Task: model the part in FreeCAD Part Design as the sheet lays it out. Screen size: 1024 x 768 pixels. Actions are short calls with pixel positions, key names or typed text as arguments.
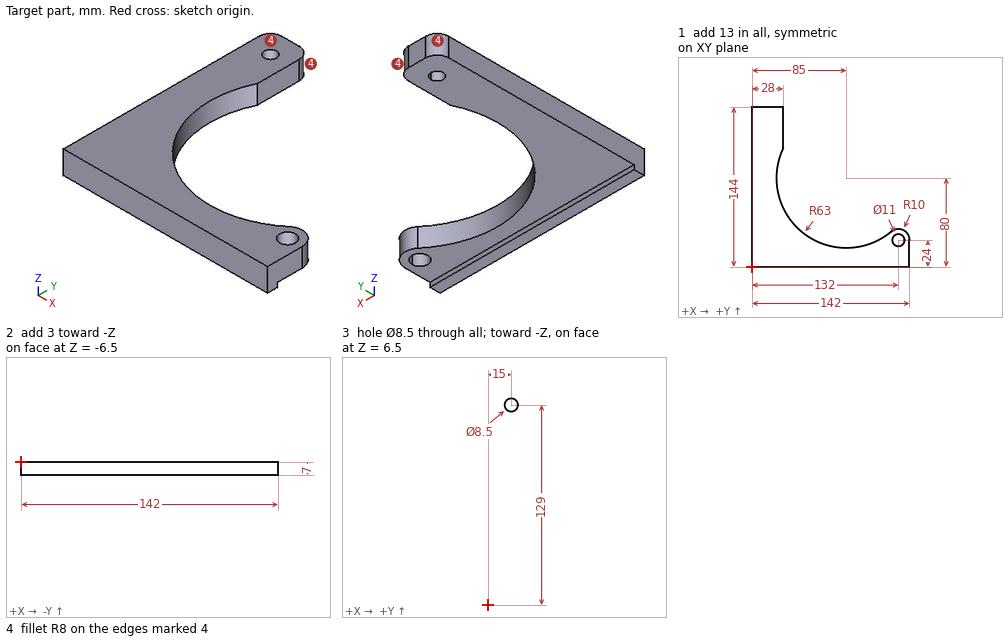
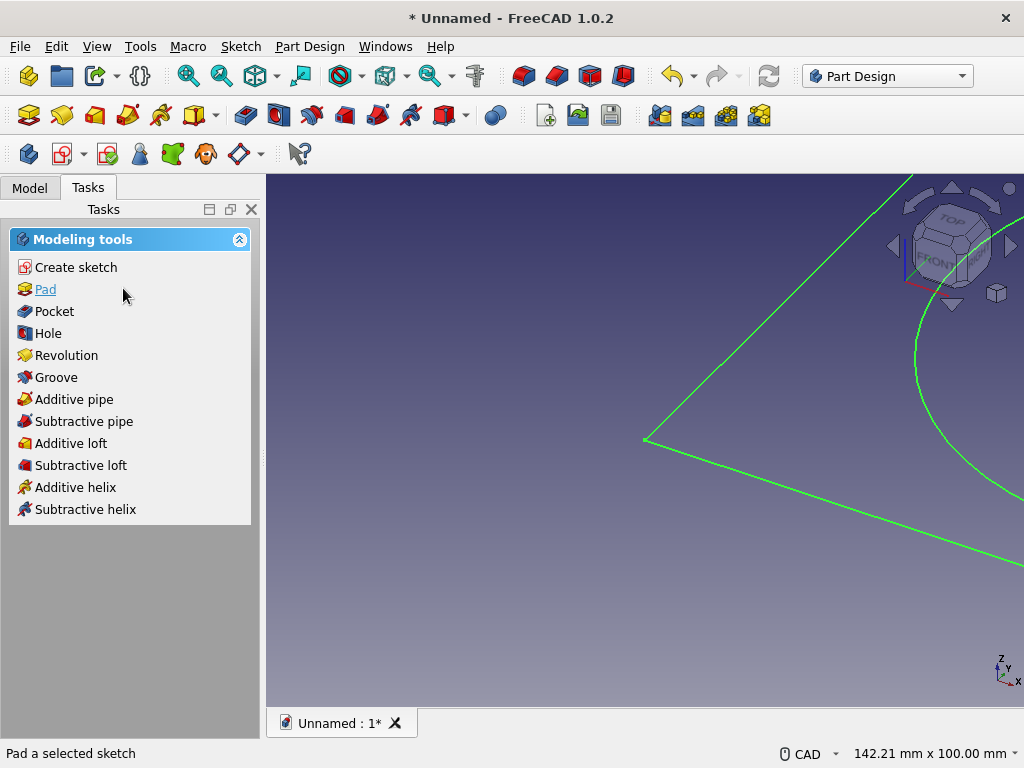
click(29, 116)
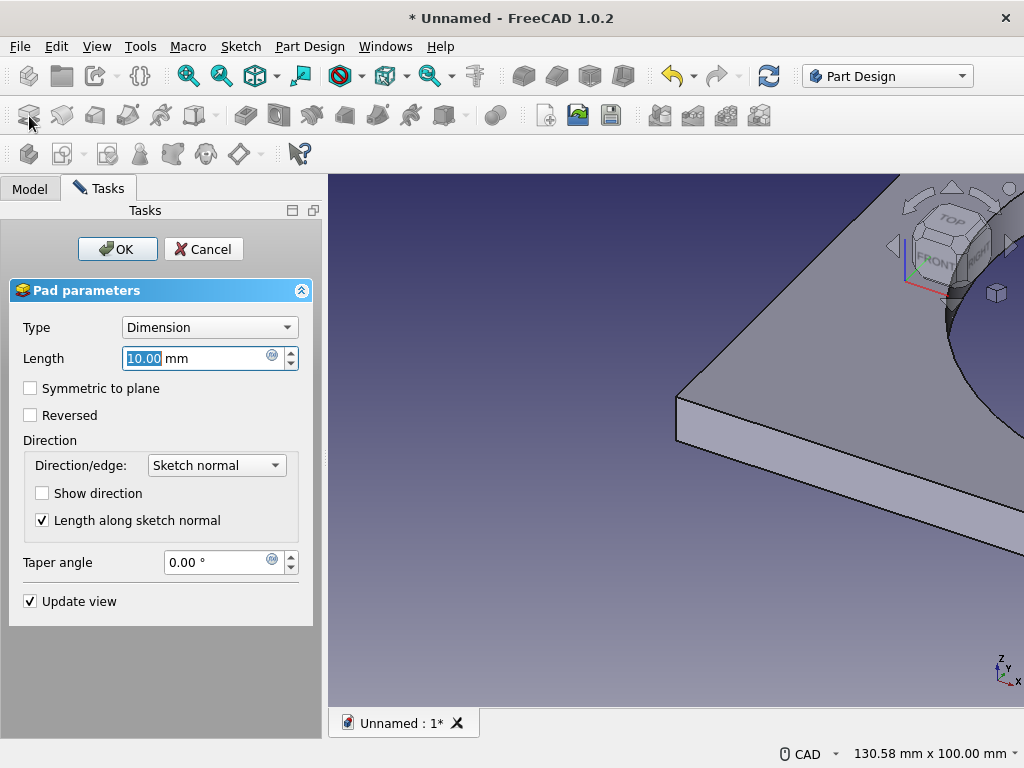
text(13)
key(Tab)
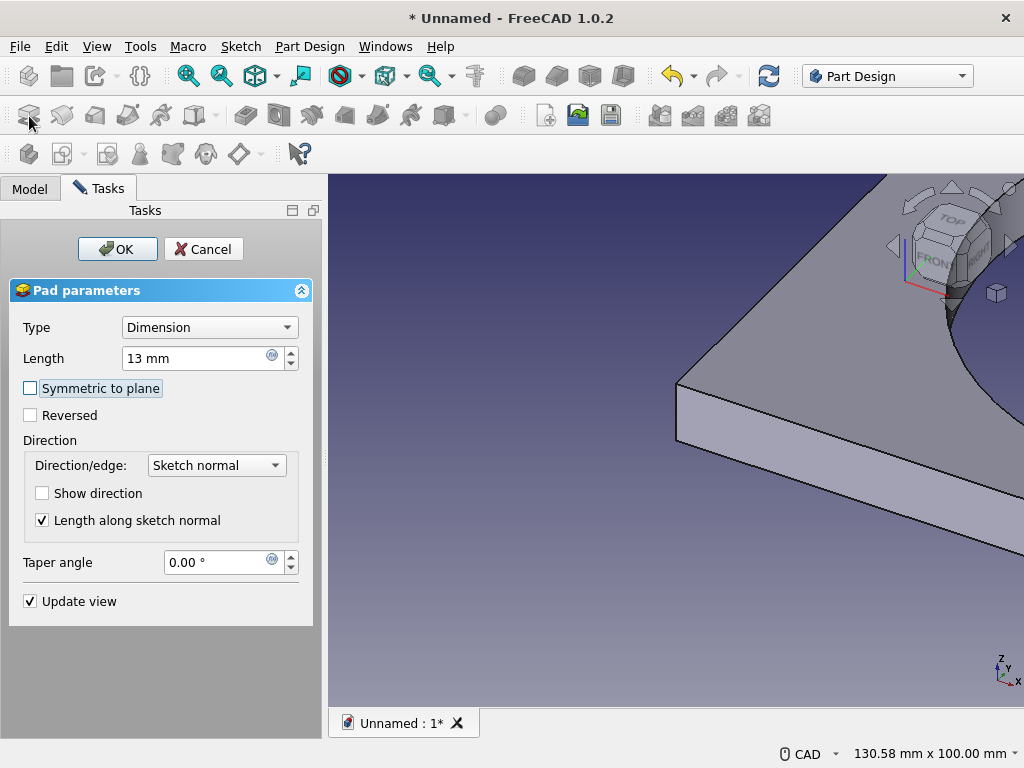
click(31, 388)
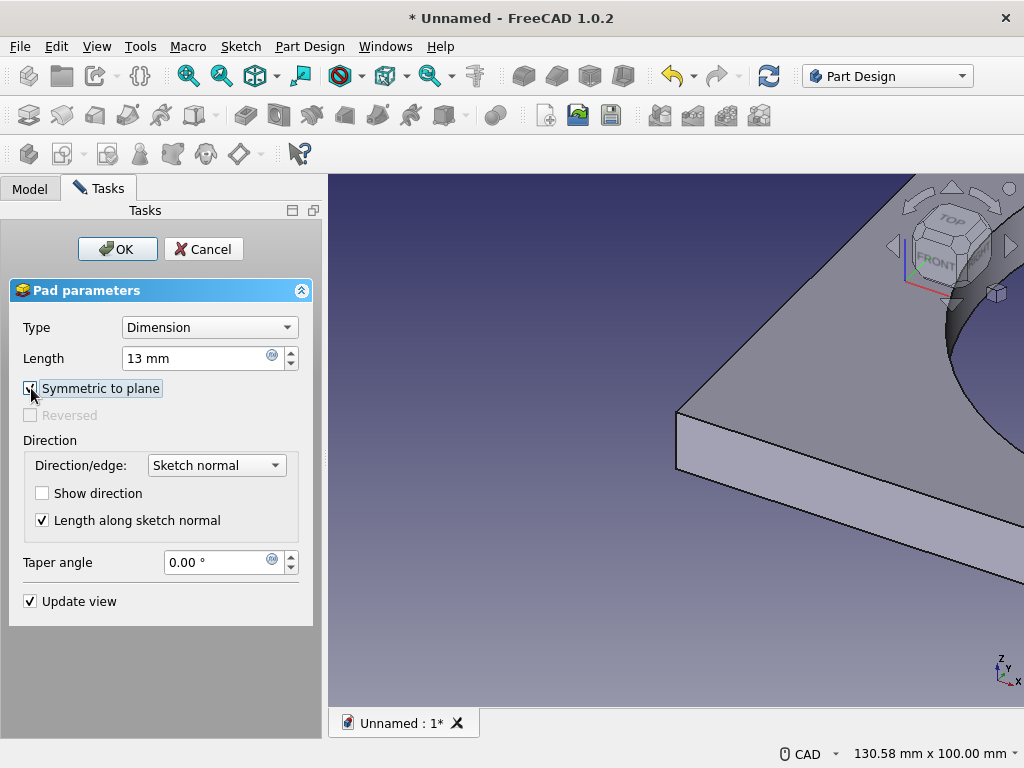
click(118, 249)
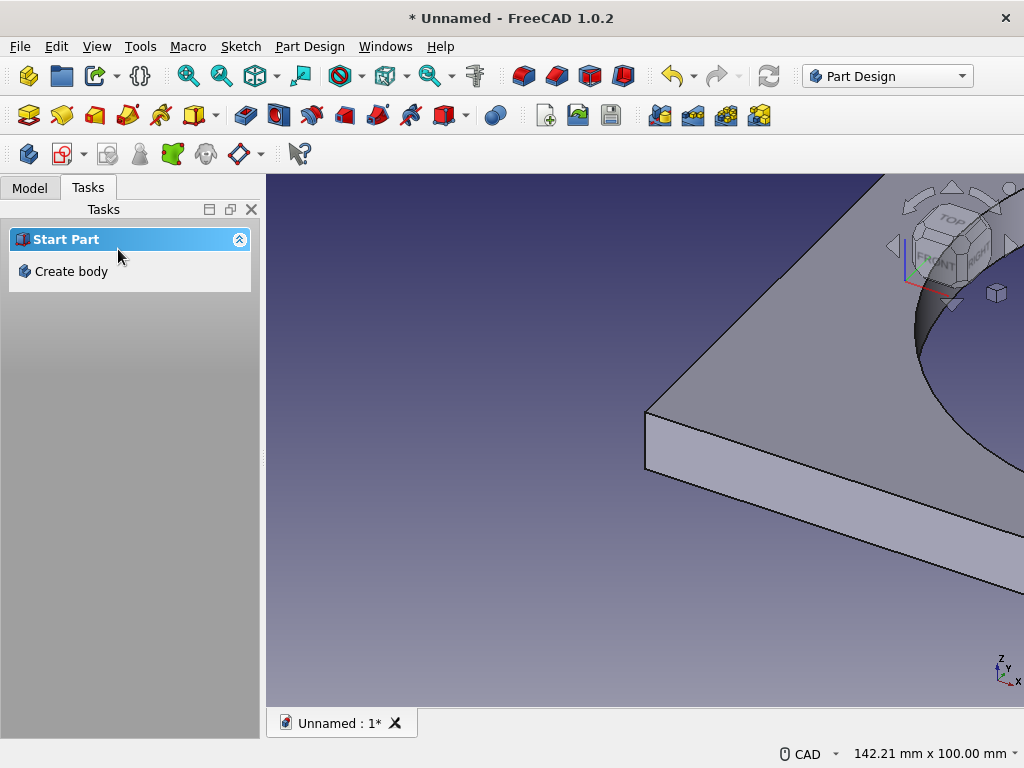
click(189, 76)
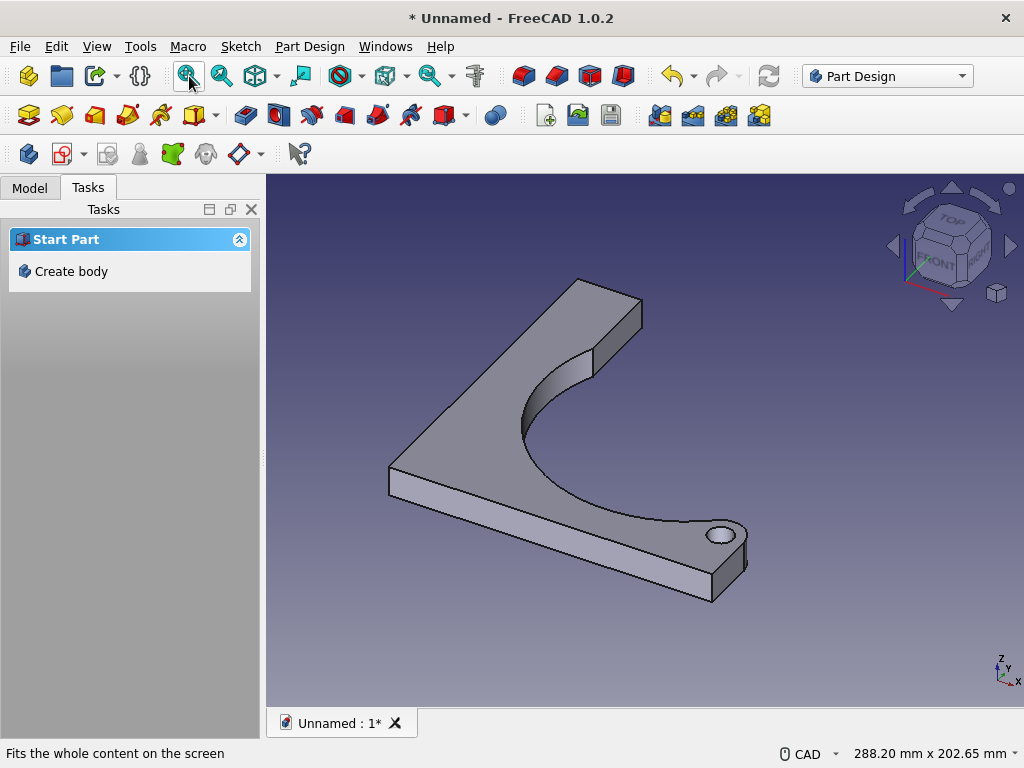
key(5)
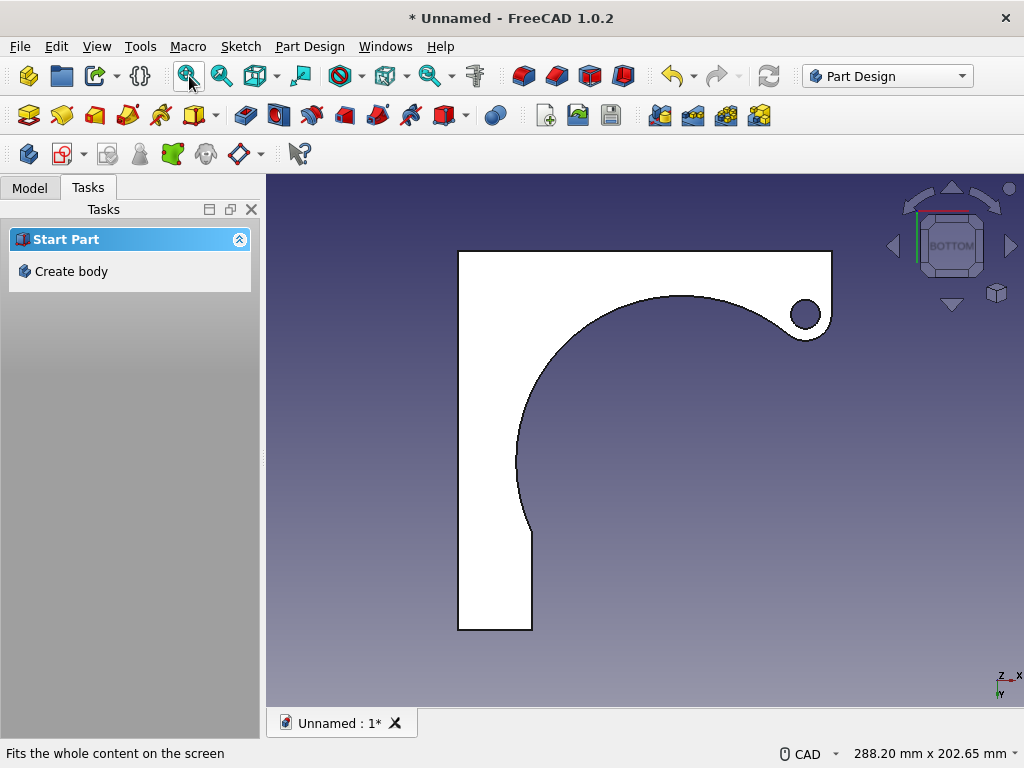
click(538, 331)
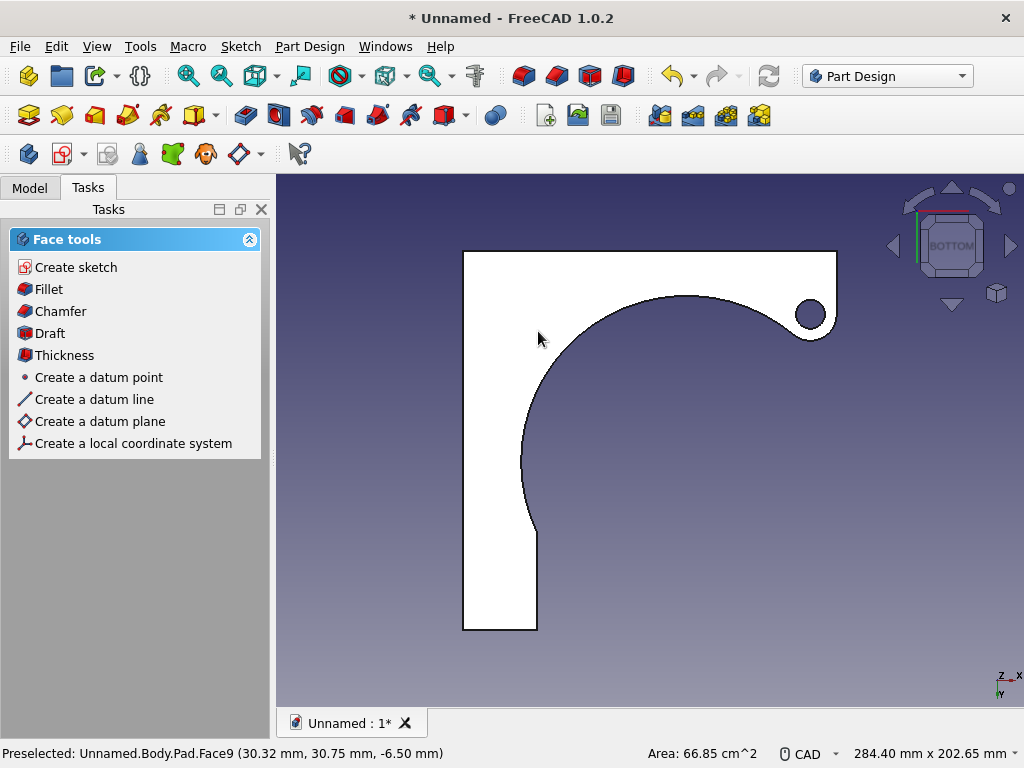
click(62, 154)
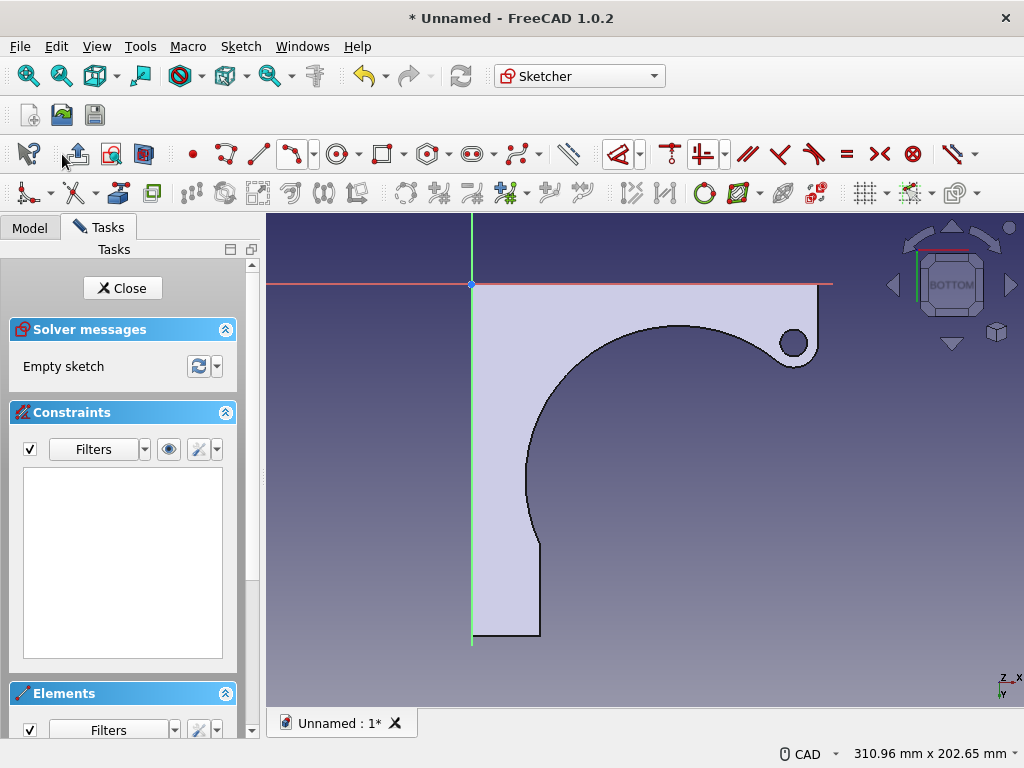
click(382, 154)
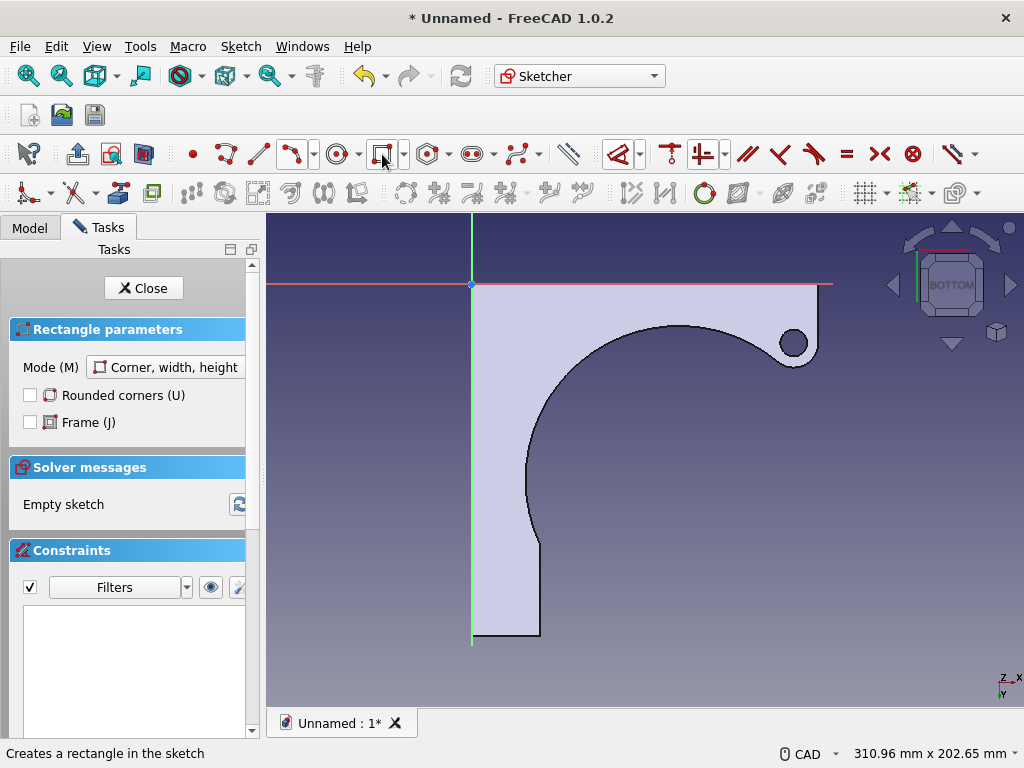
click(472, 284)
move(818, 302)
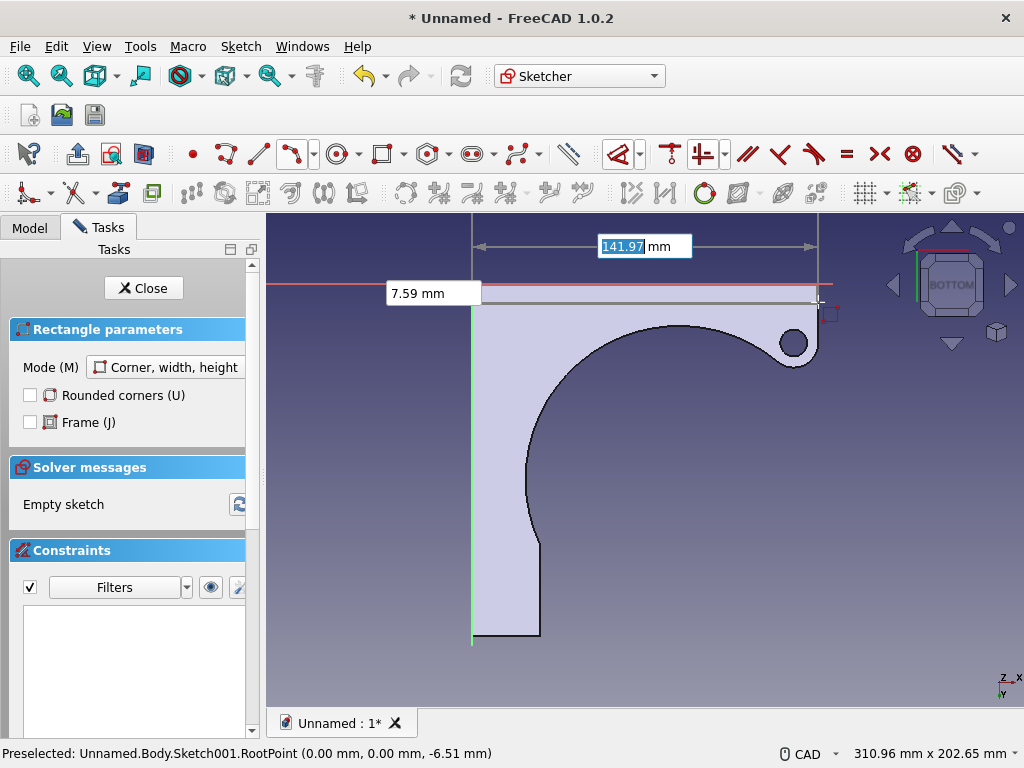
text(142)
key(Tab)
text(7)
key(Return)
key(Escape)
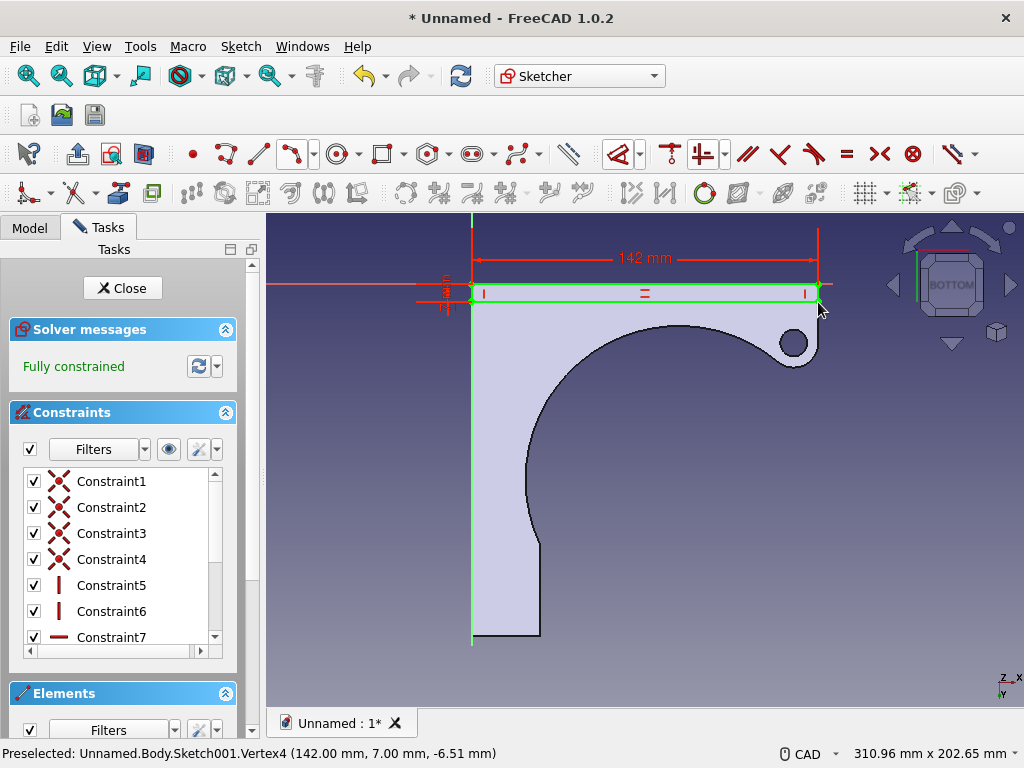
click(123, 288)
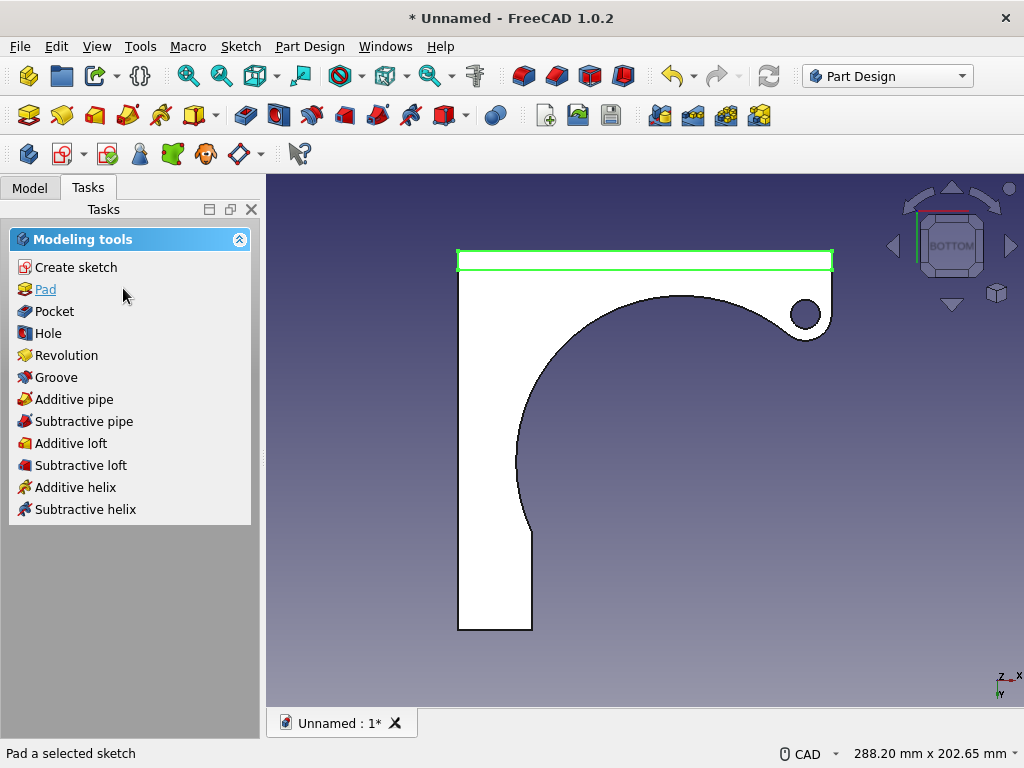
click(29, 116)